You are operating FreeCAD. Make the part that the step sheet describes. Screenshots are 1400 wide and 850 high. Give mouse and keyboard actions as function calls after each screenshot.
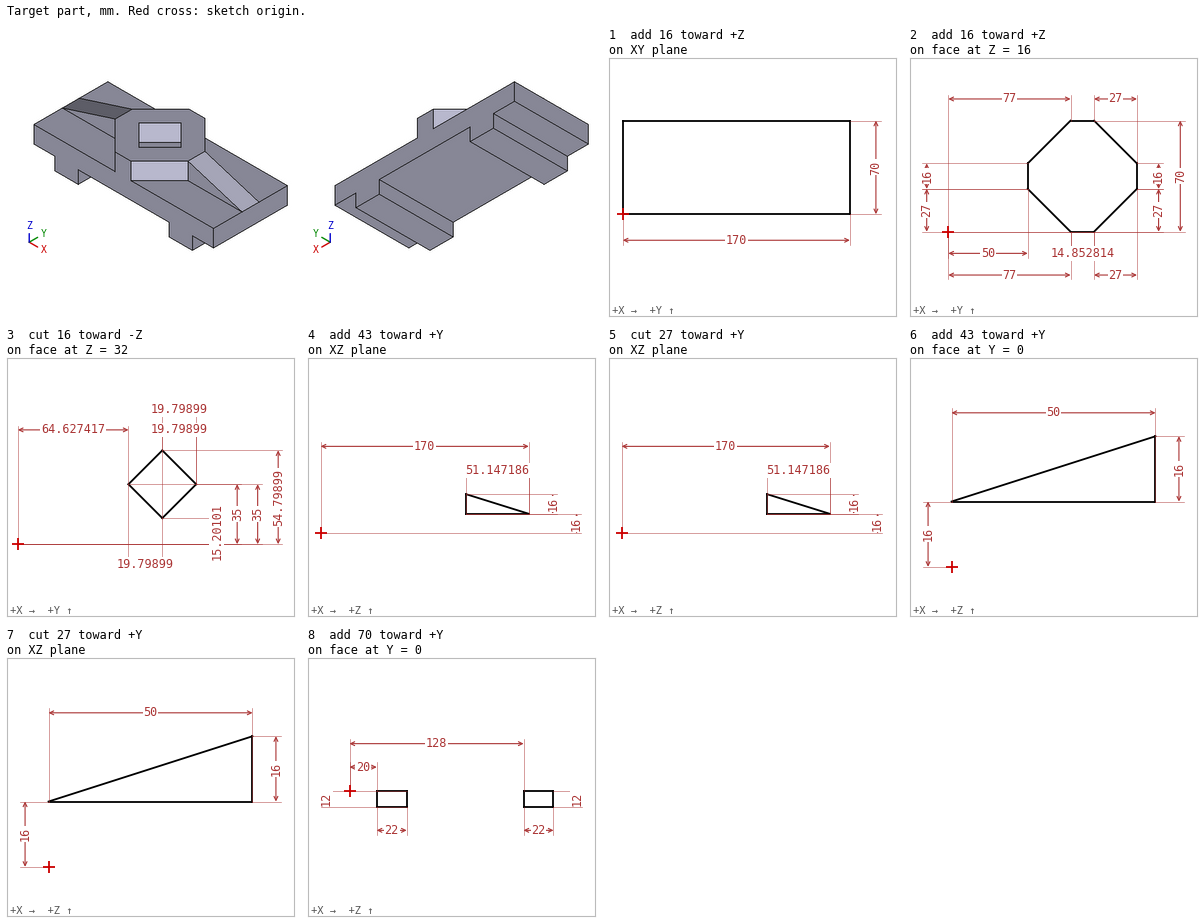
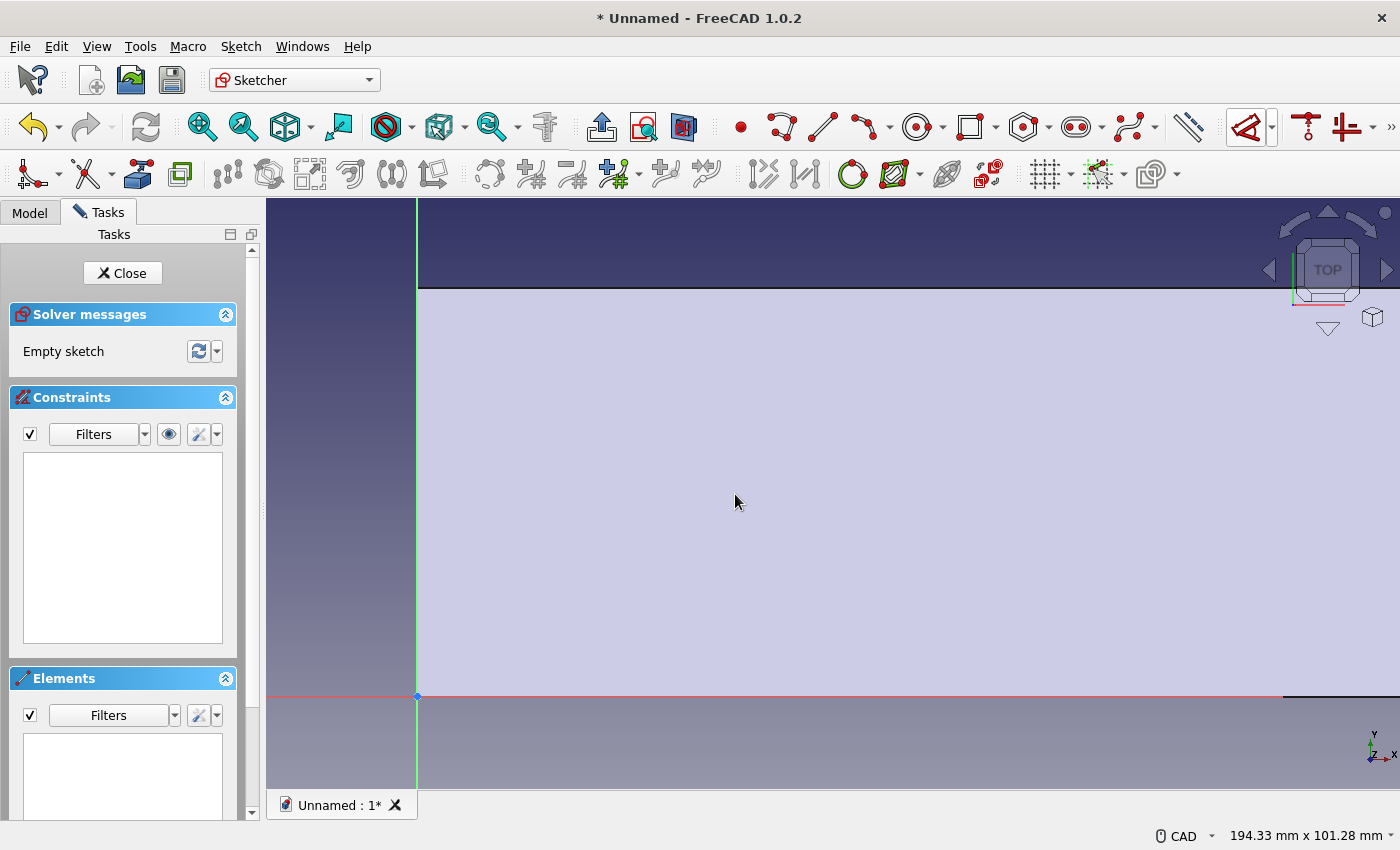
key(g)
key(m)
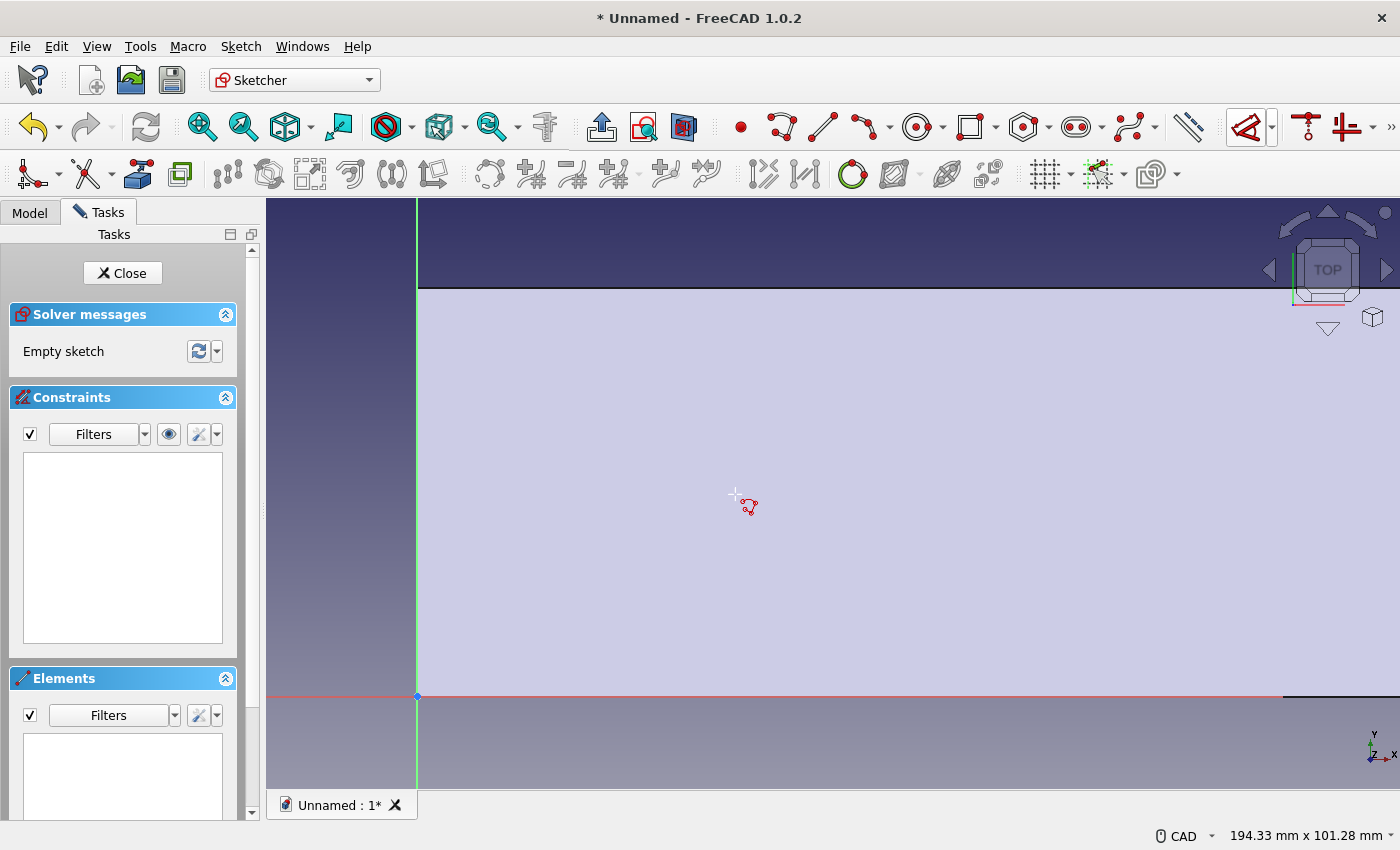
click(709, 539)
click(867, 697)
click(953, 688)
click(1111, 539)
click(1111, 446)
click(953, 288)
click(867, 288)
click(709, 446)
click(709, 540)
key(Escape)
key(Escape)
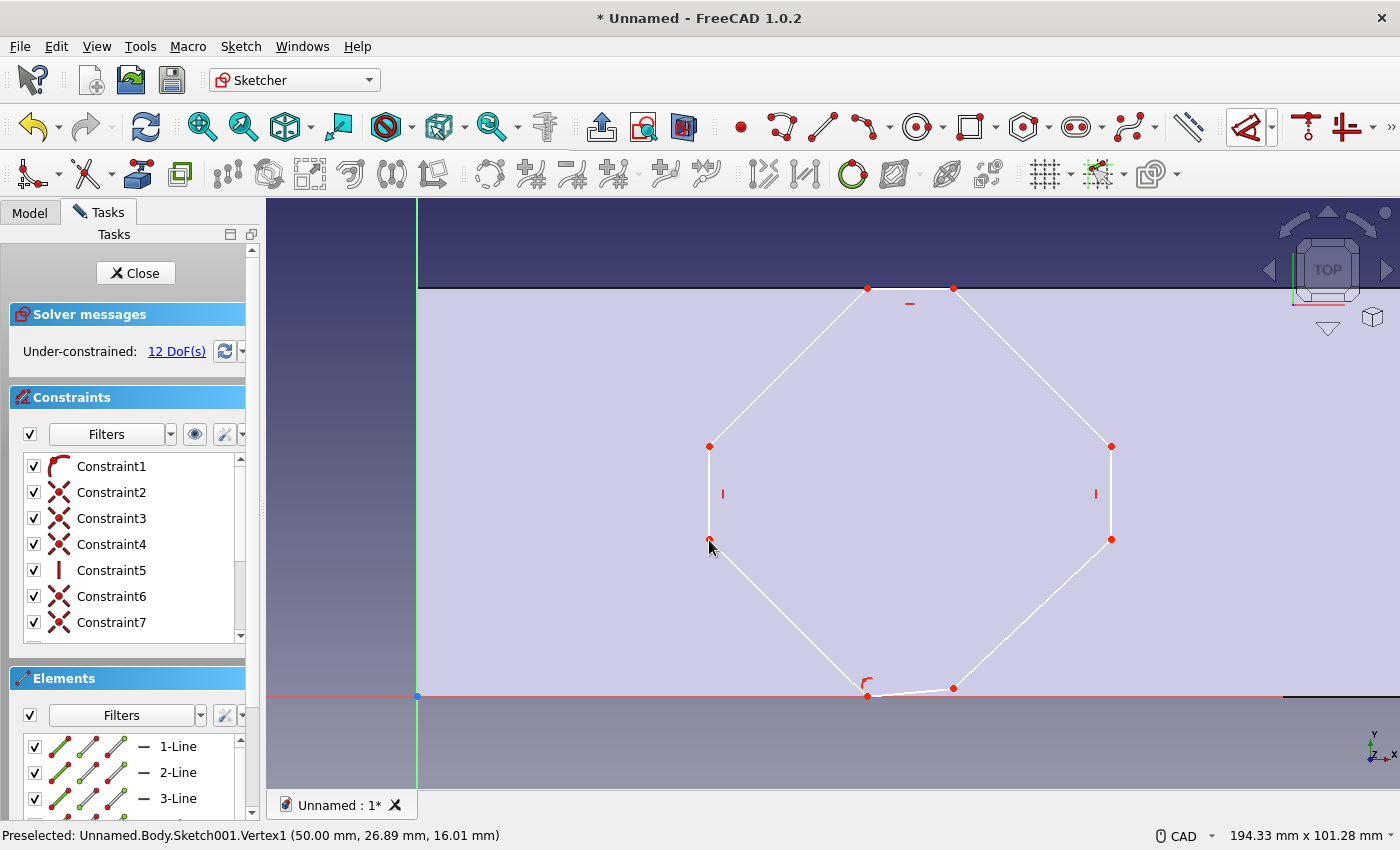
click(893, 695)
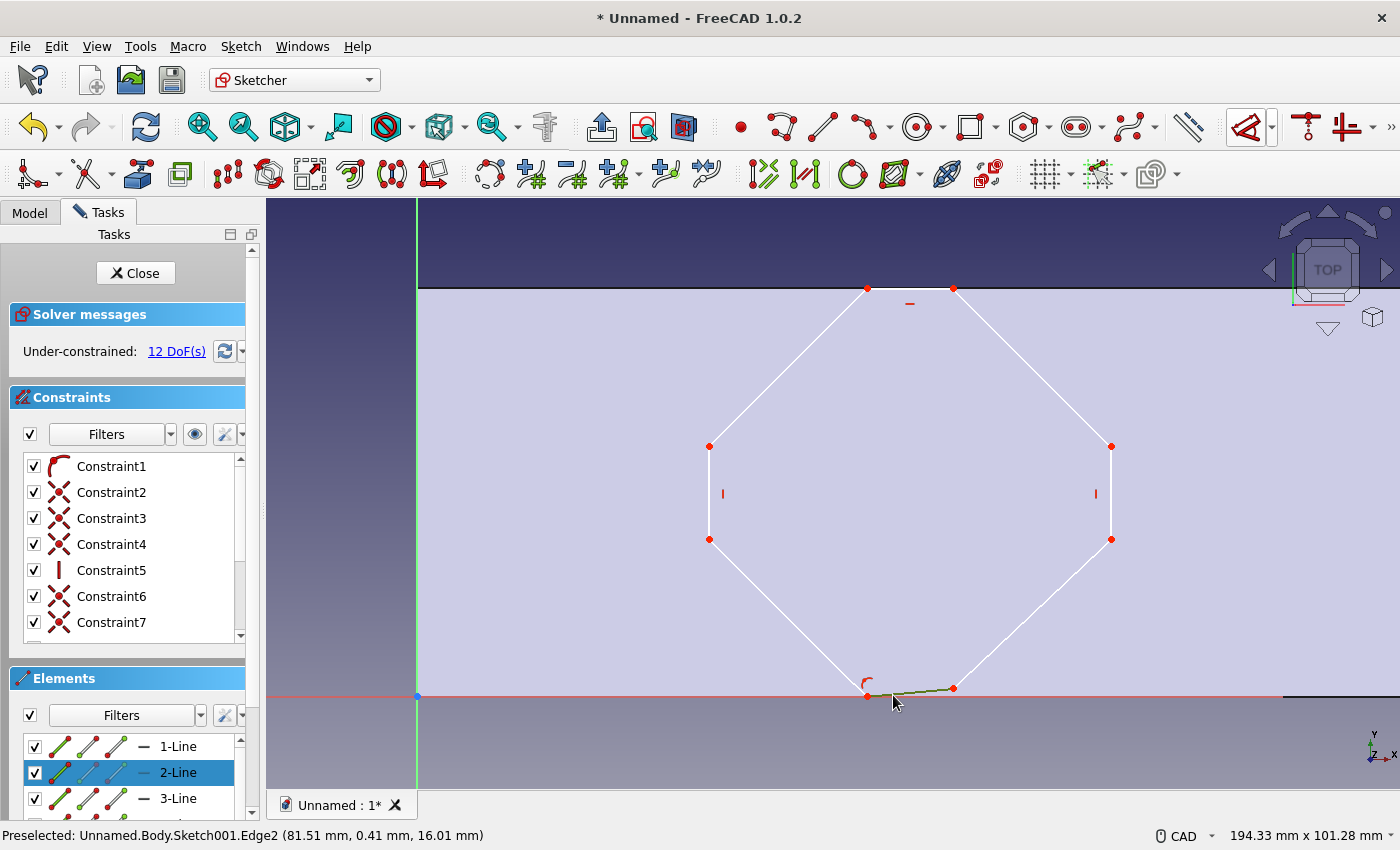
key(h)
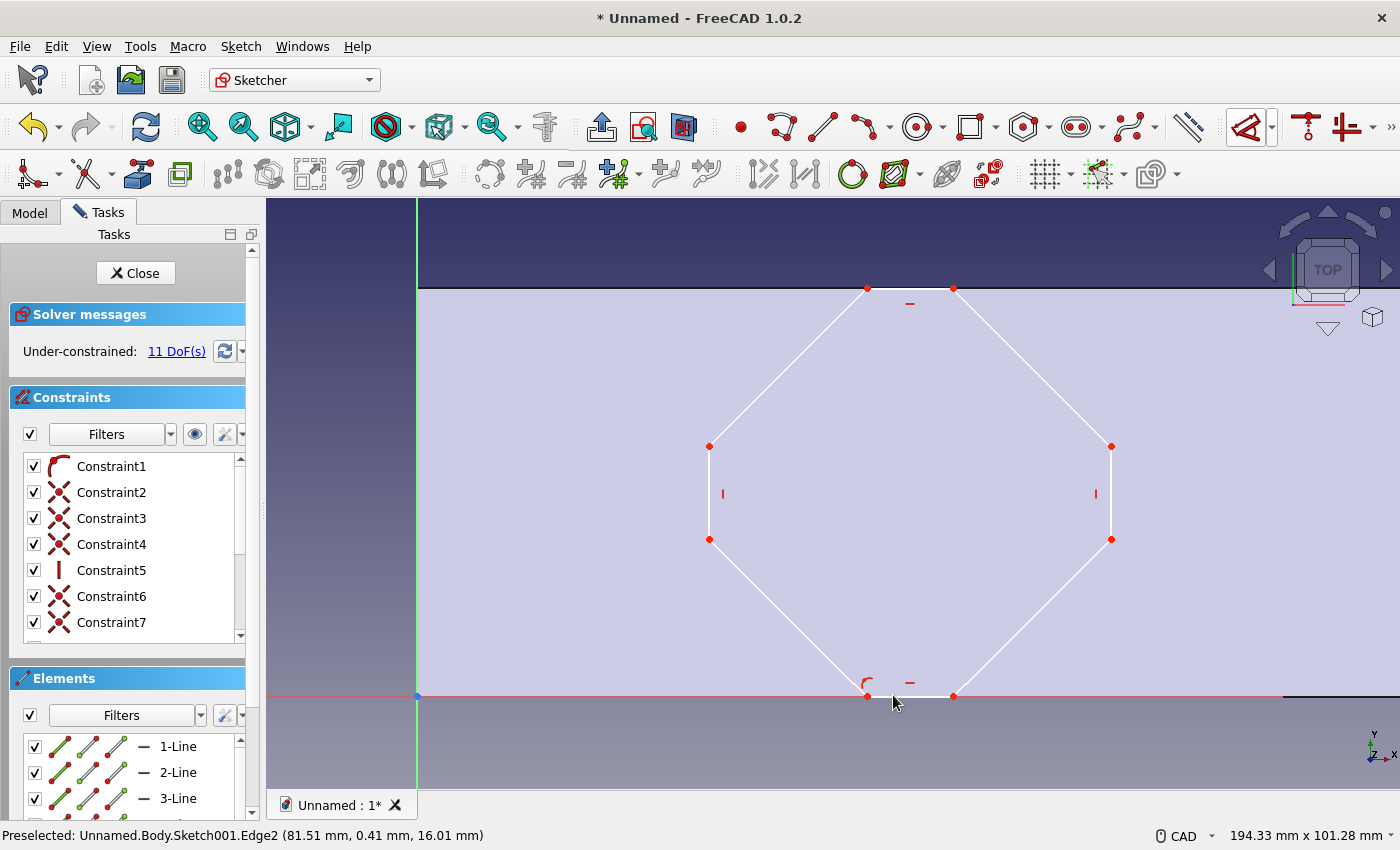
key(d)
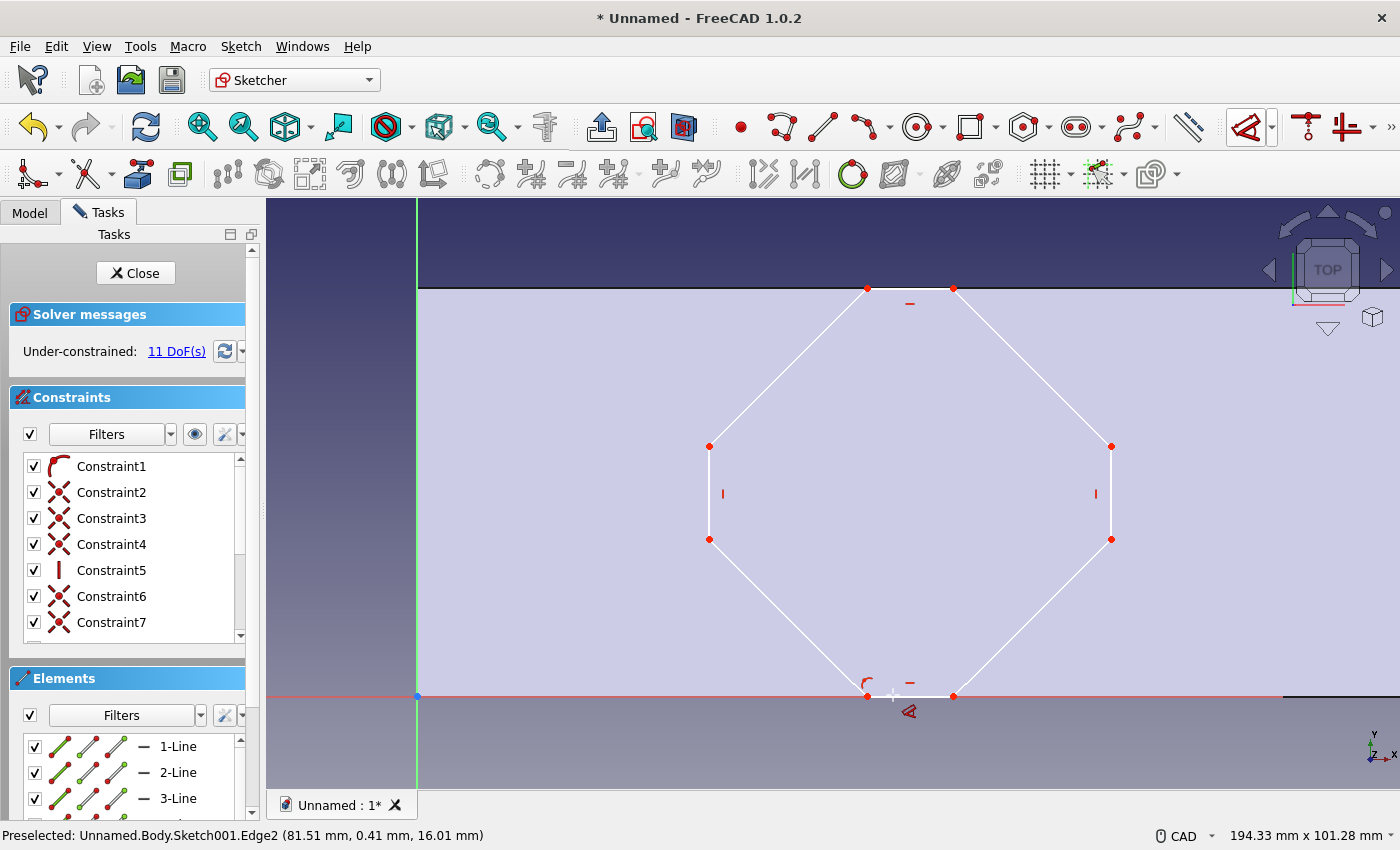
click(1111, 512)
click(1145, 493)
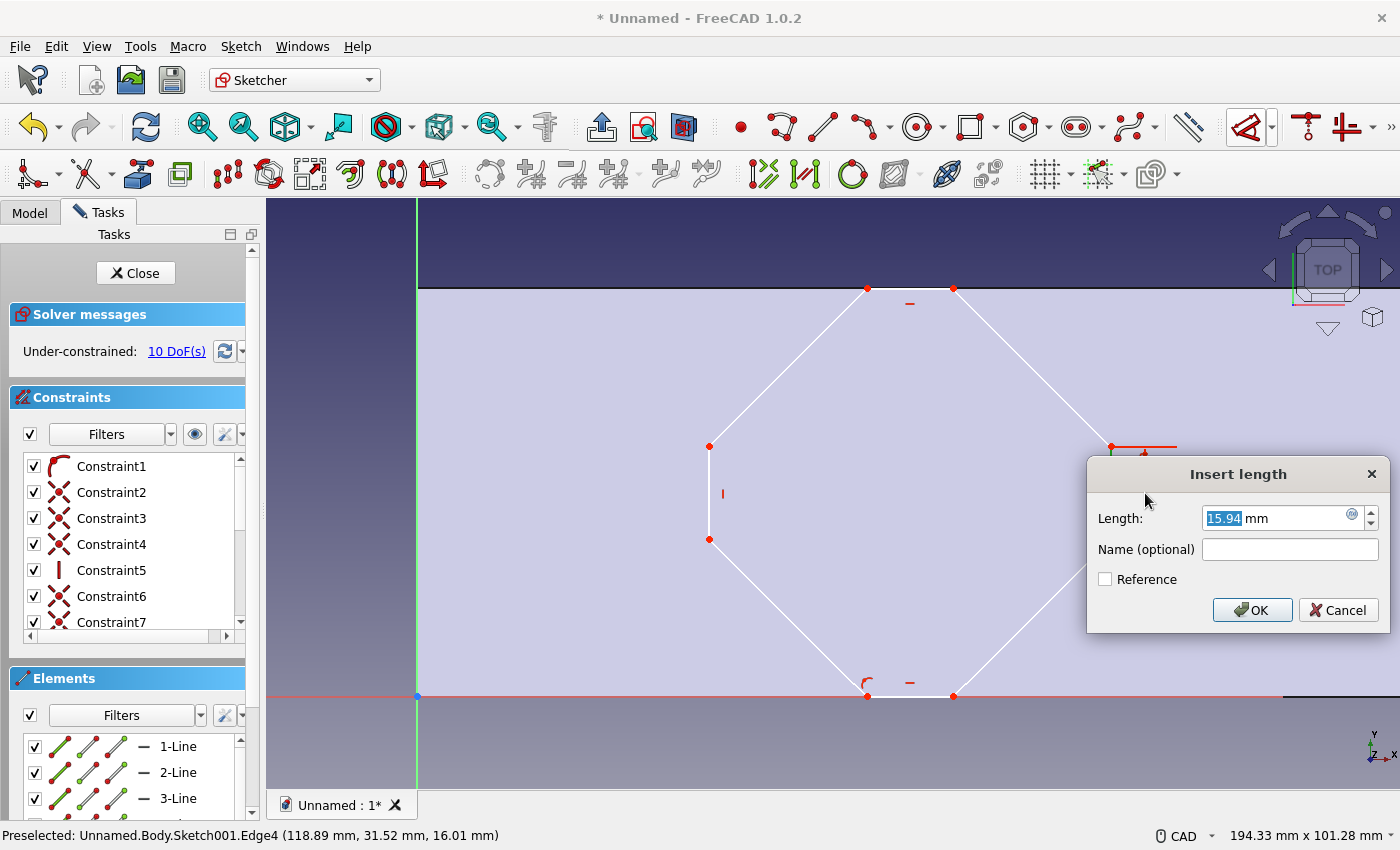
text(16)
key(Return)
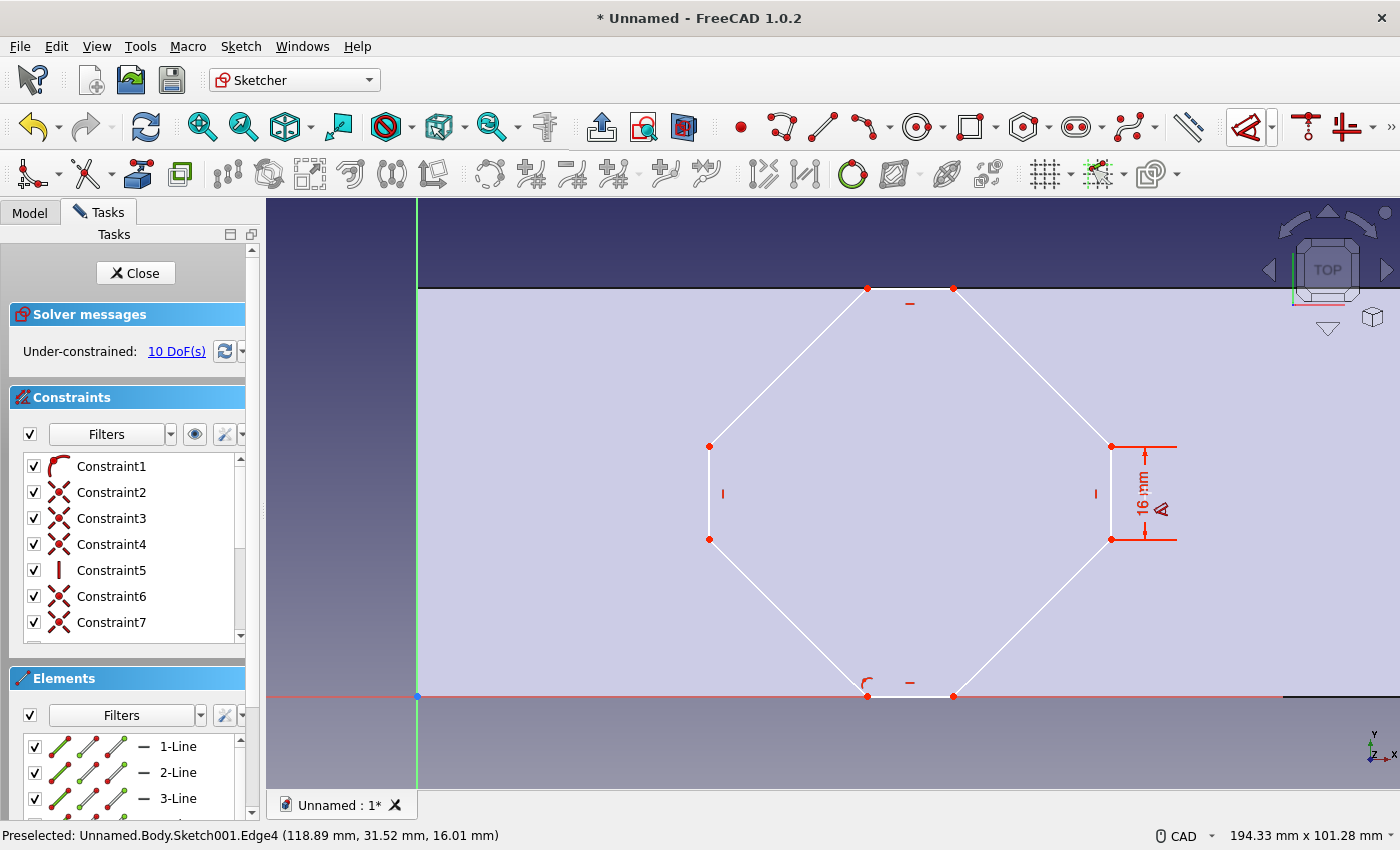
click(709, 475)
click(675, 493)